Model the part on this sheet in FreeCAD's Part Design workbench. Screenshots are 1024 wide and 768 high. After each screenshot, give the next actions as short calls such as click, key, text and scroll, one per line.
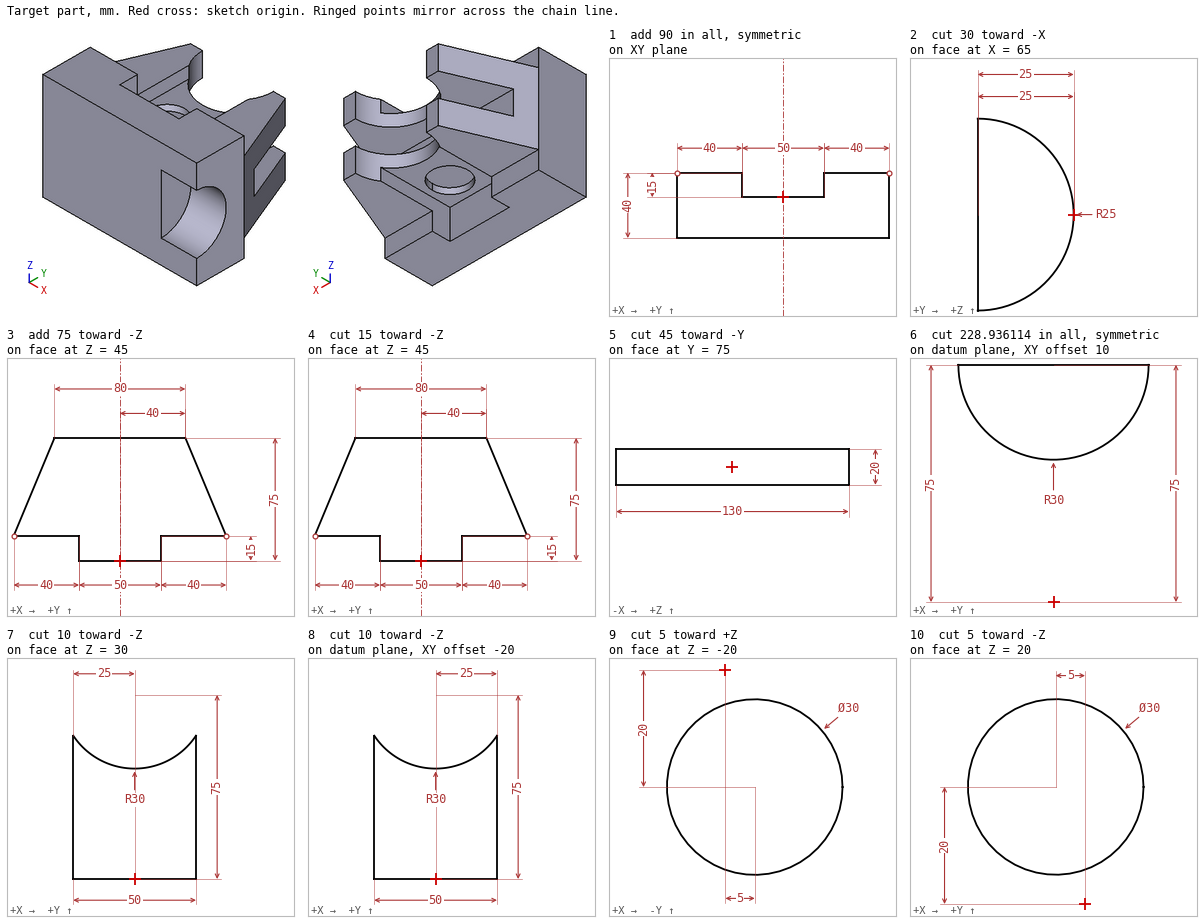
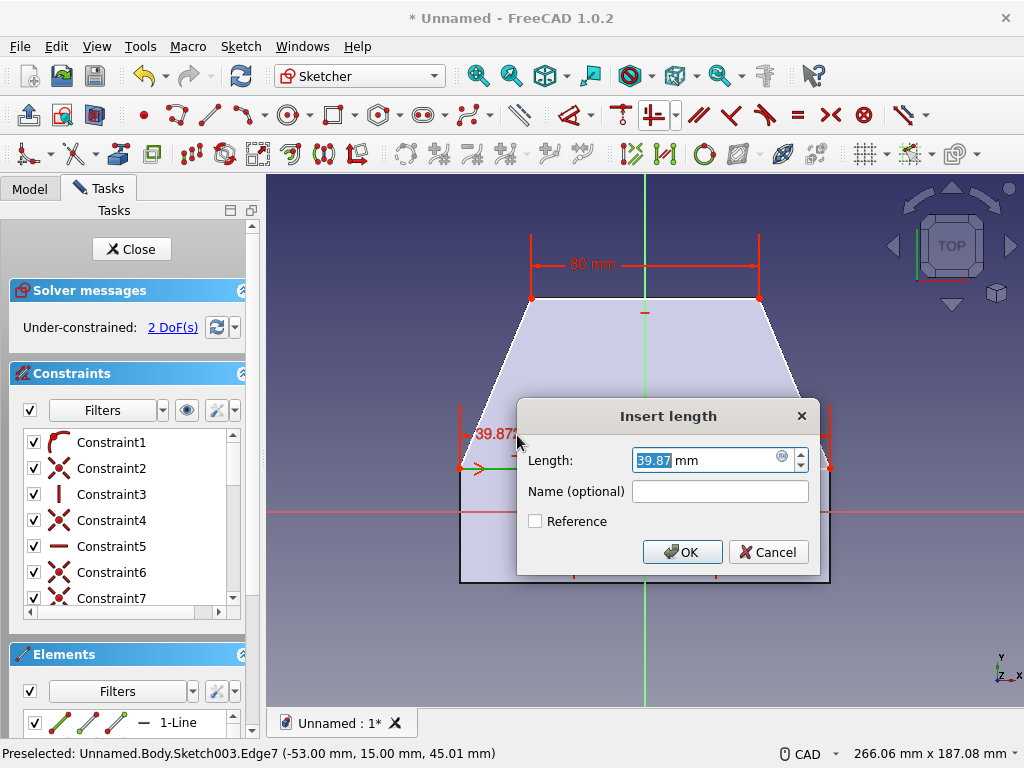
text(40)
key(Return)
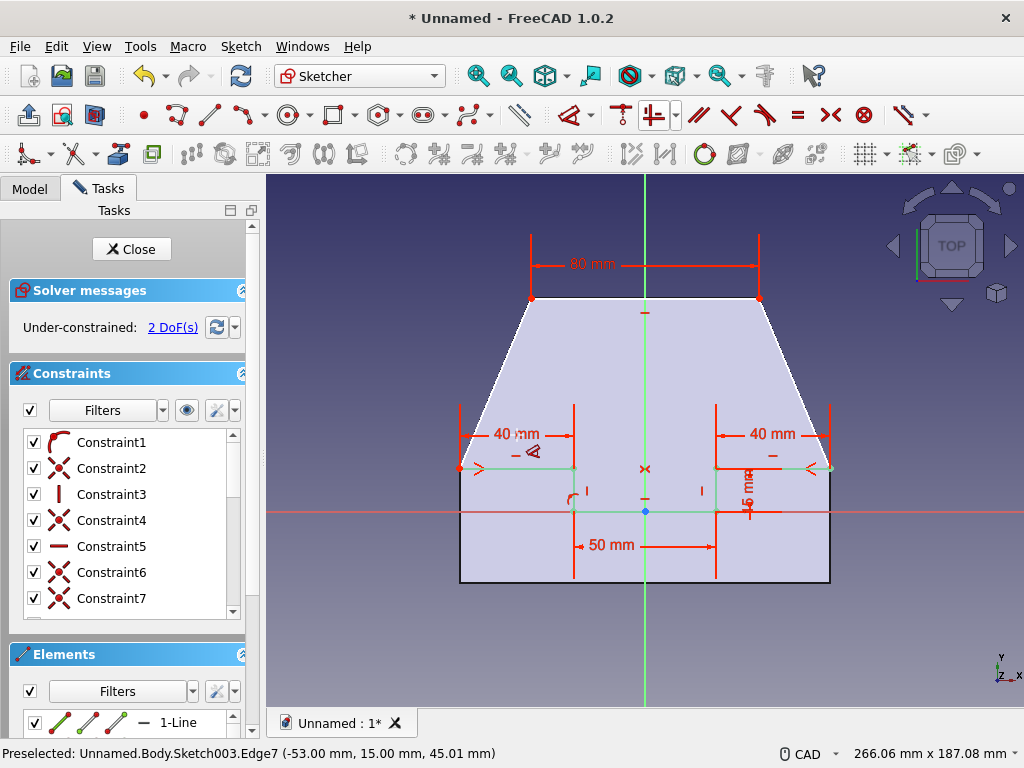
click(759, 299)
click(702, 546)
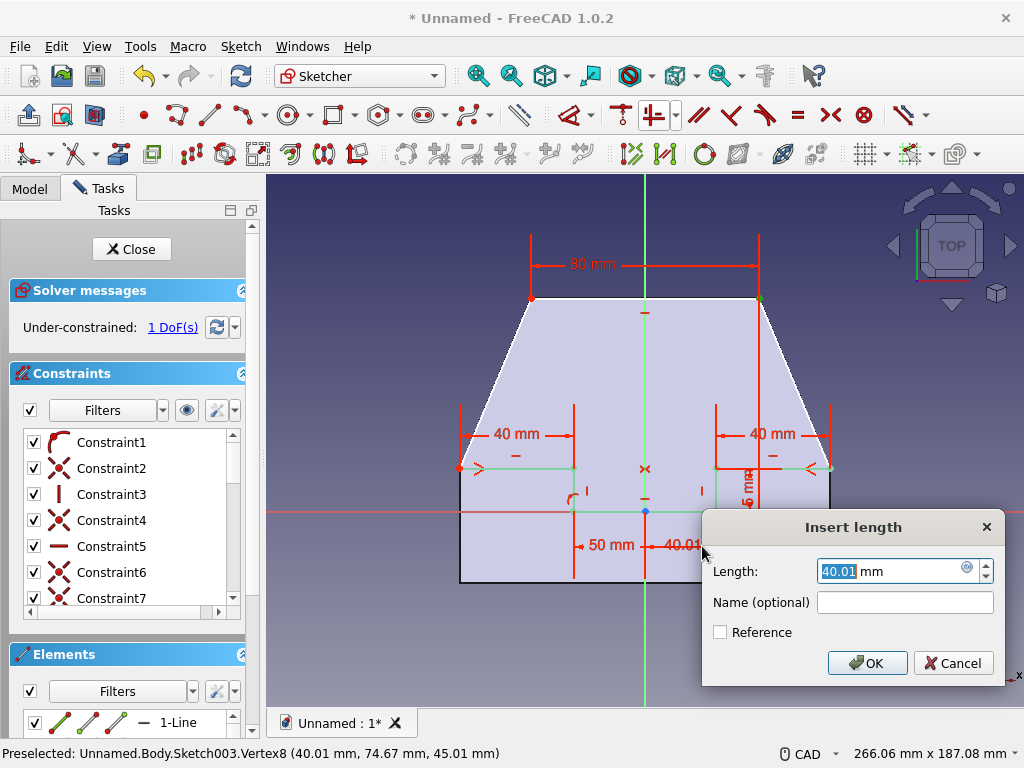
text(40)
key(Return)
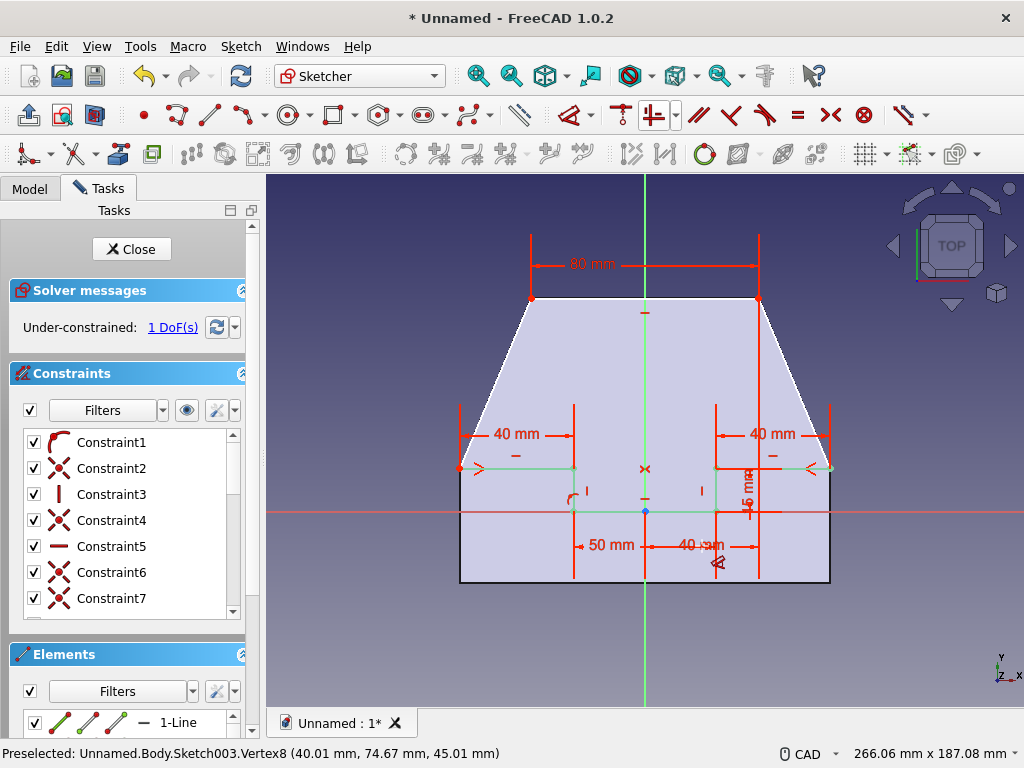
click(759, 299)
click(793, 331)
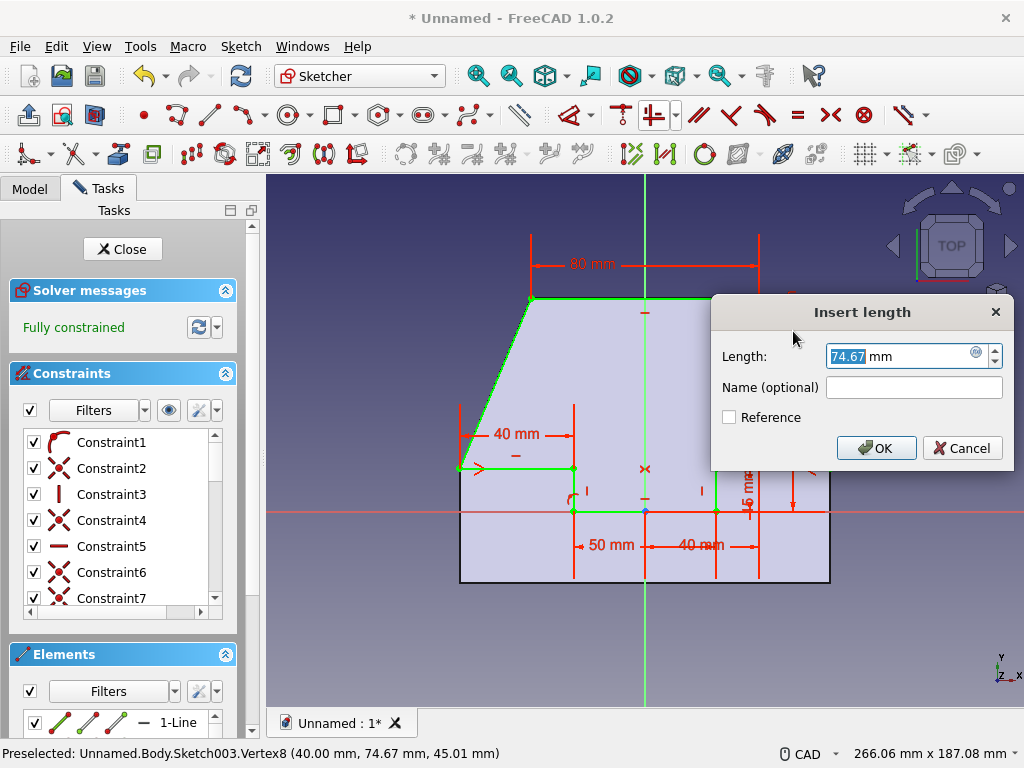
text(75)
key(Return)
key(Escape)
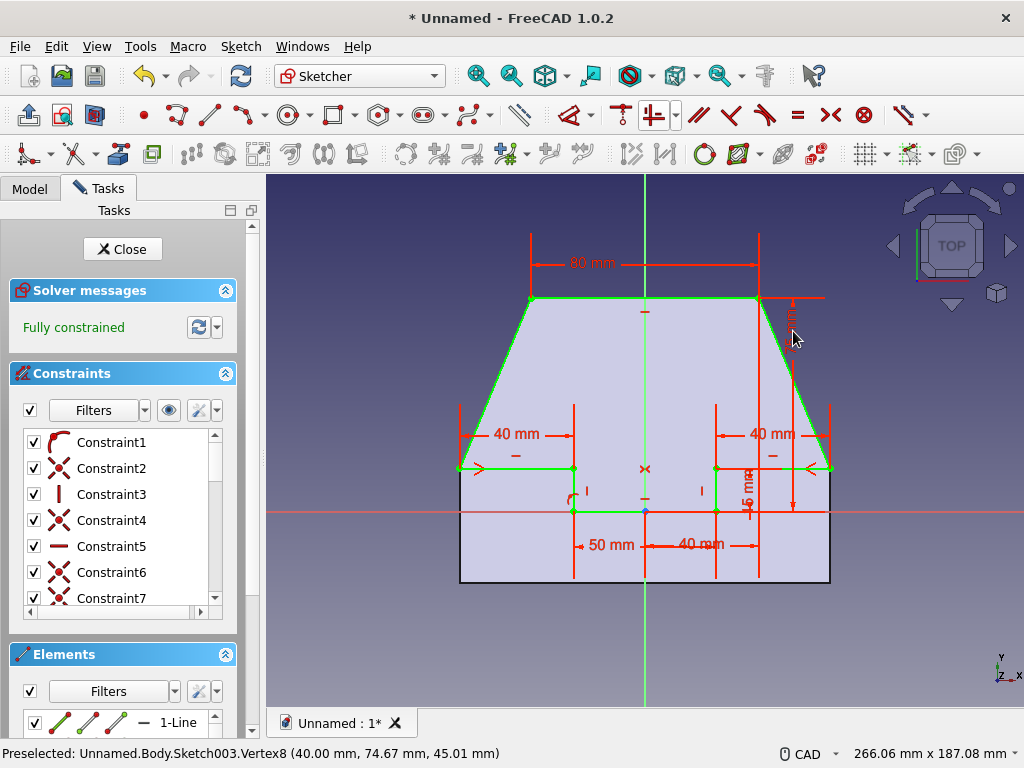
click(123, 249)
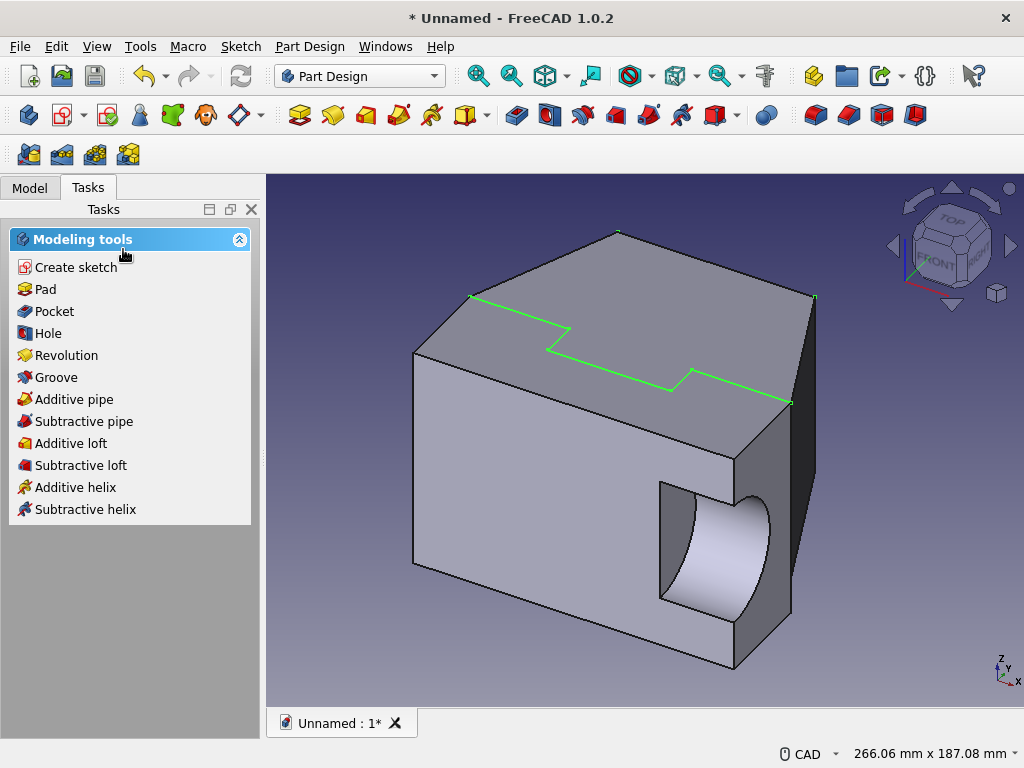
click(517, 116)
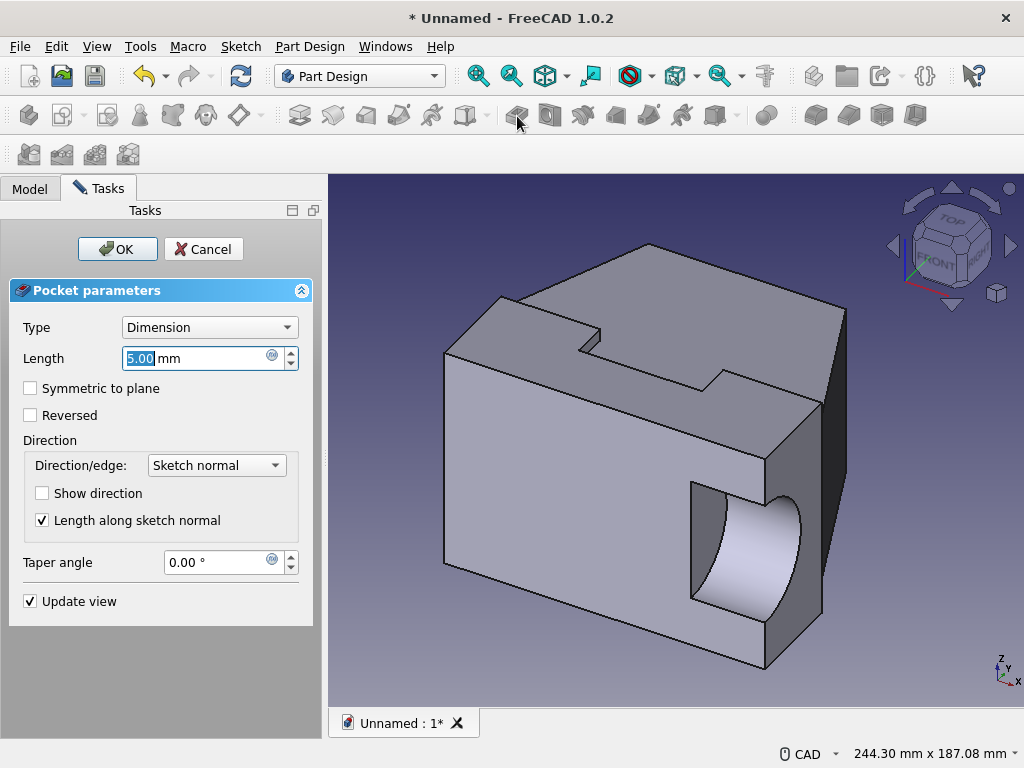
text(15)
key(Tab)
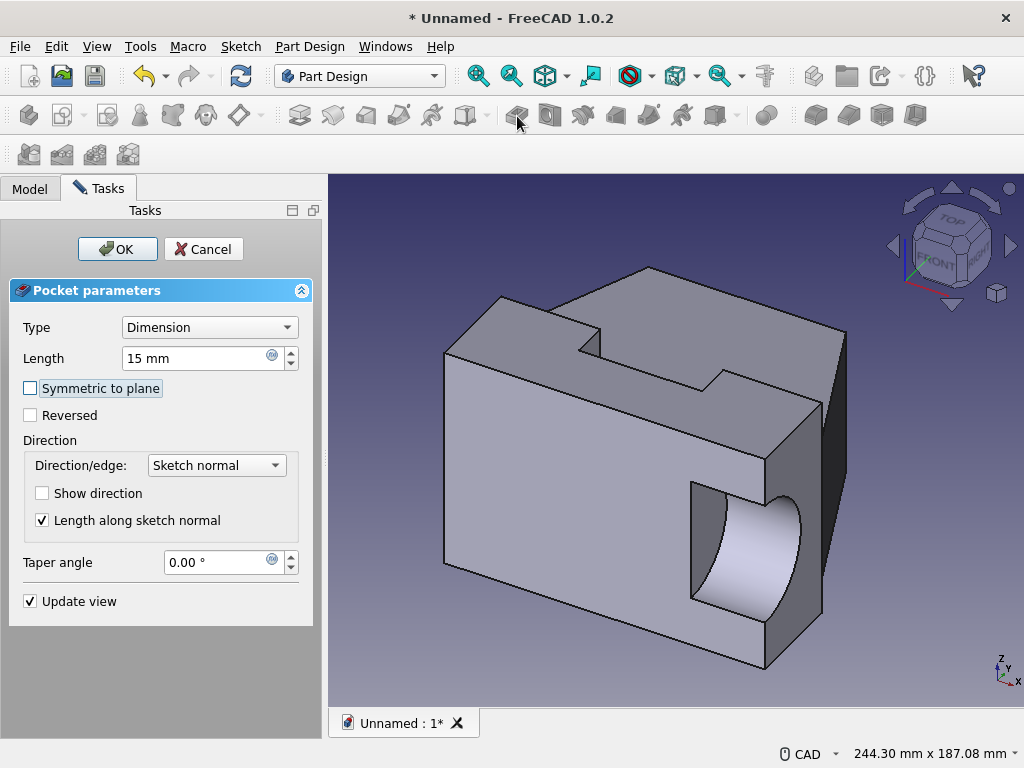
click(118, 249)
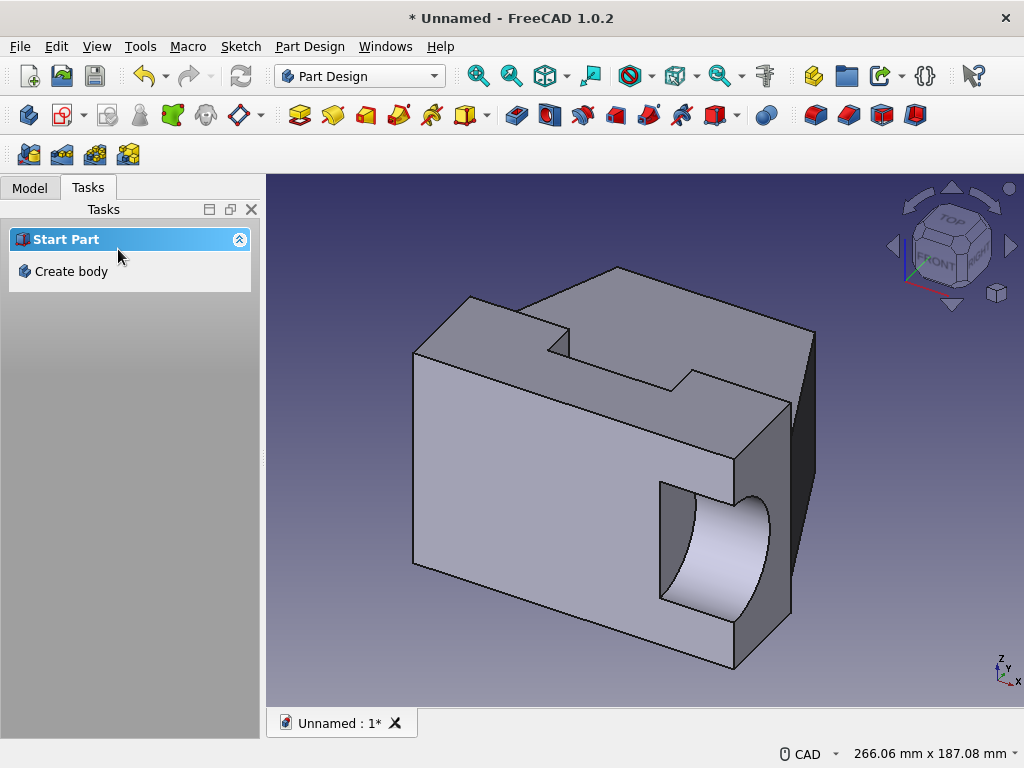
key(4)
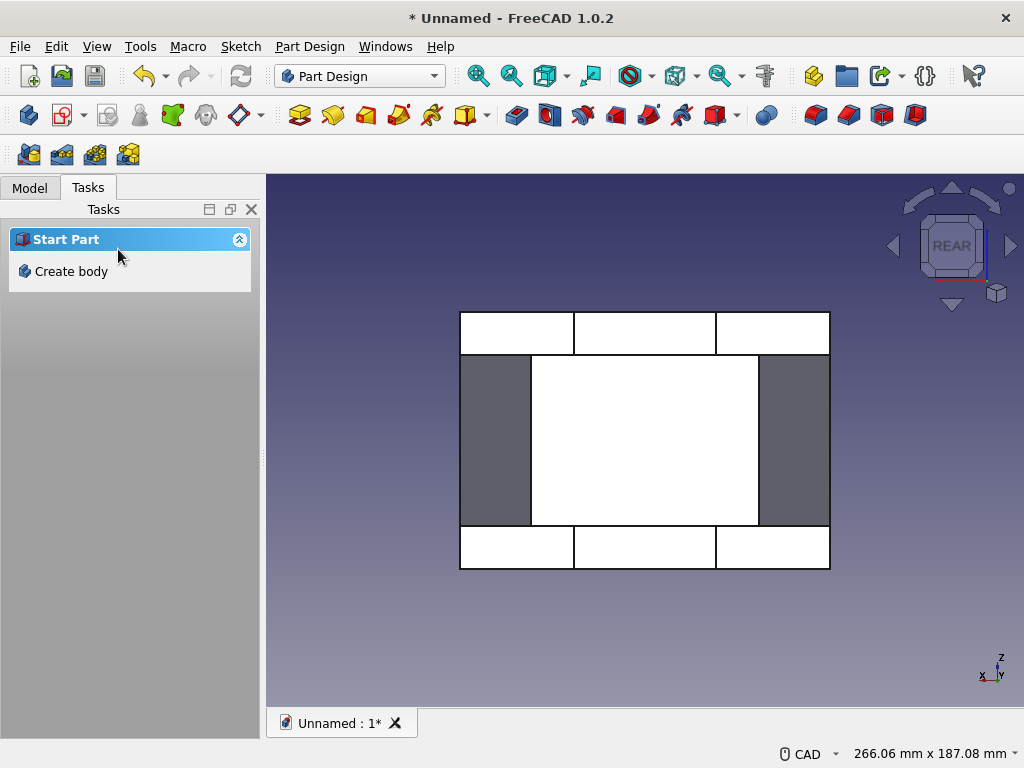
click(645, 439)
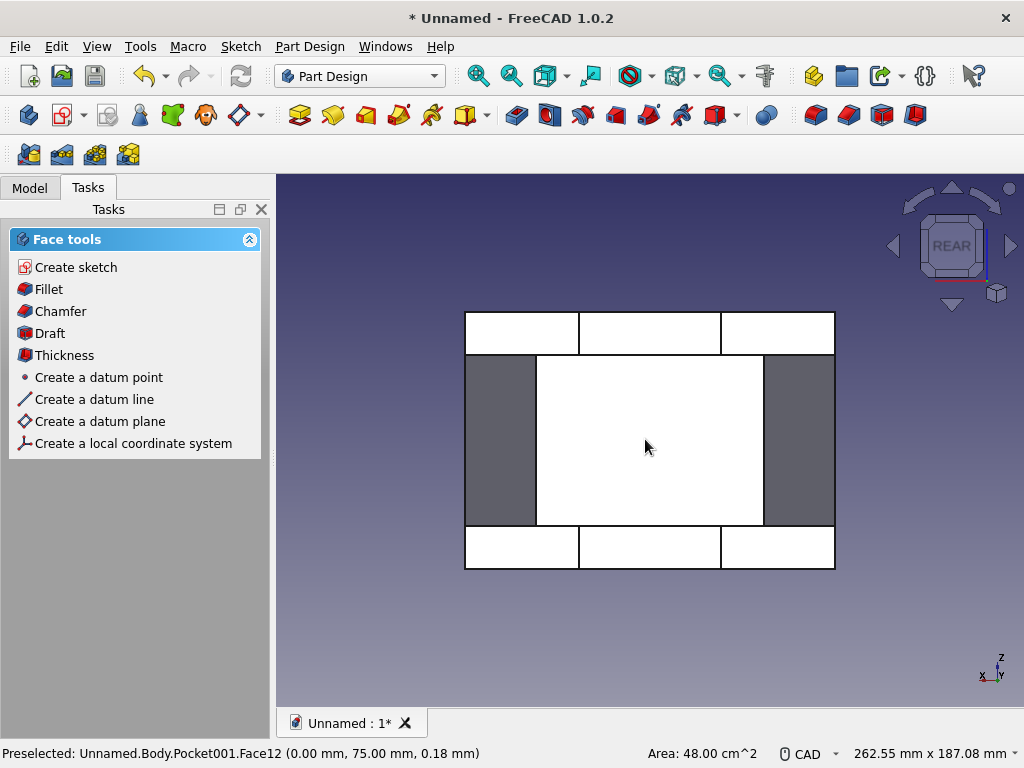
click(62, 116)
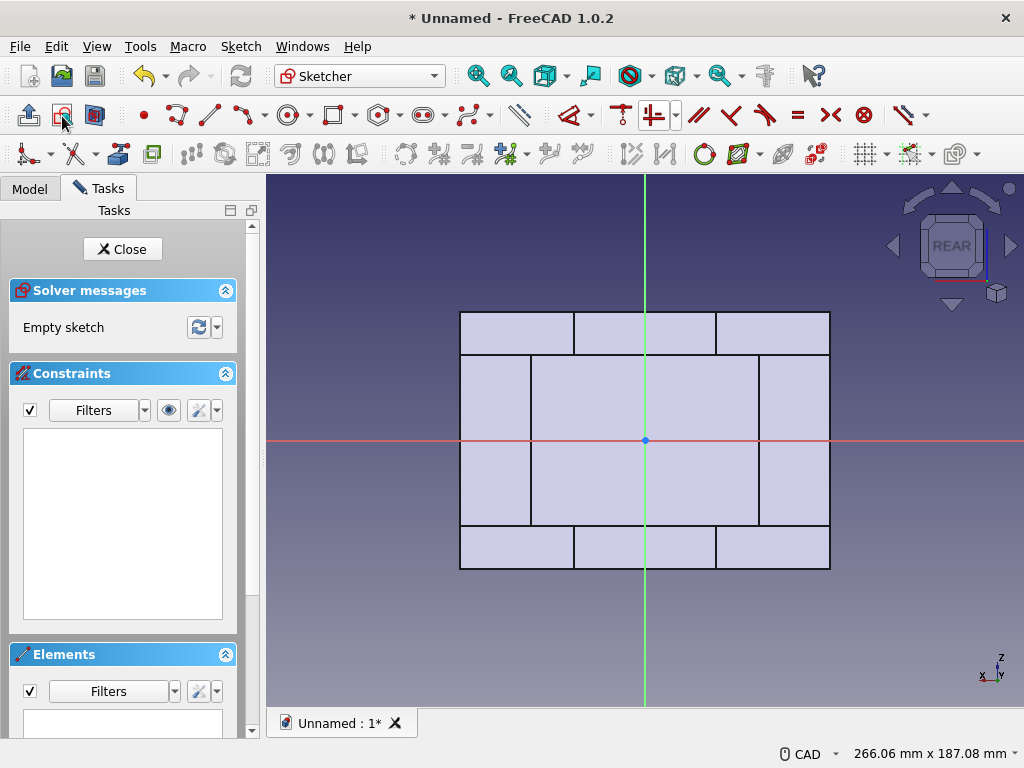
key(g)
key(v)